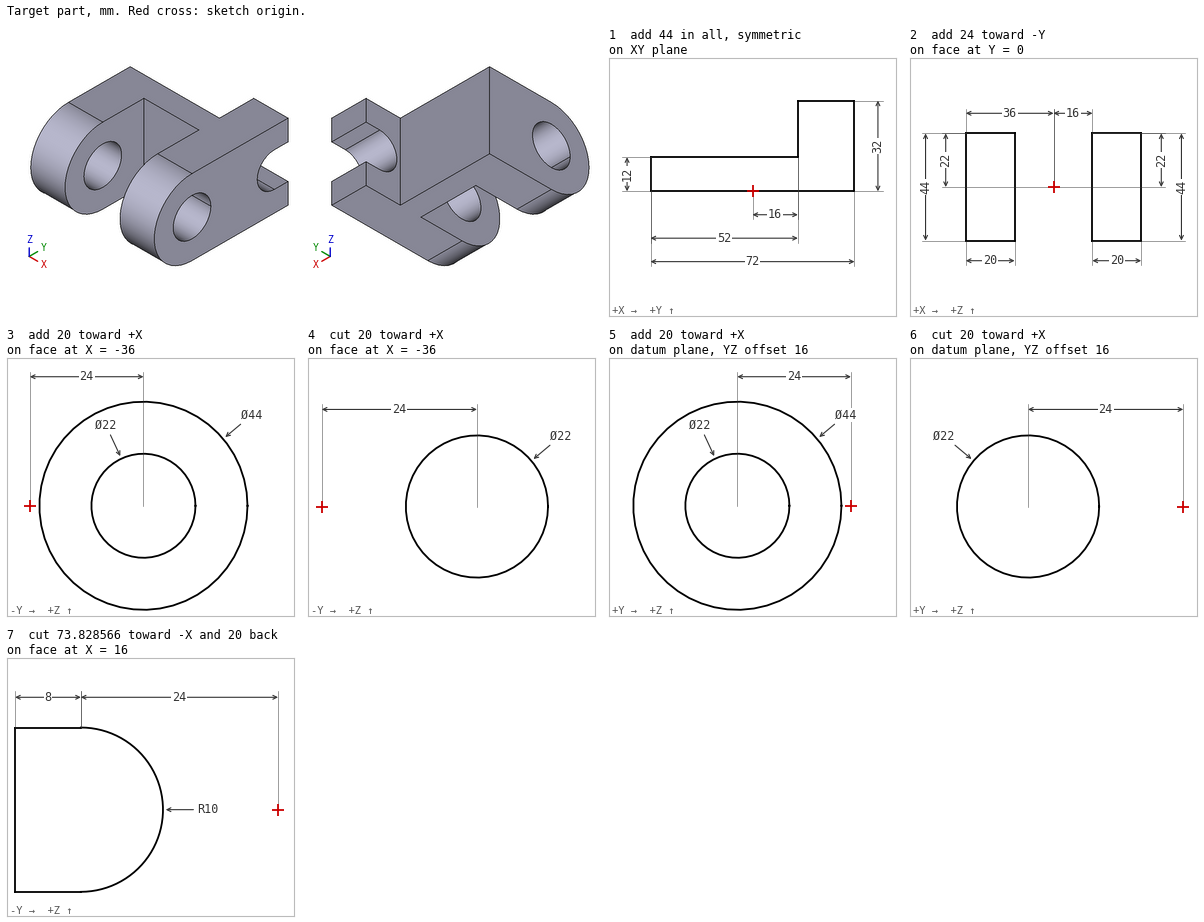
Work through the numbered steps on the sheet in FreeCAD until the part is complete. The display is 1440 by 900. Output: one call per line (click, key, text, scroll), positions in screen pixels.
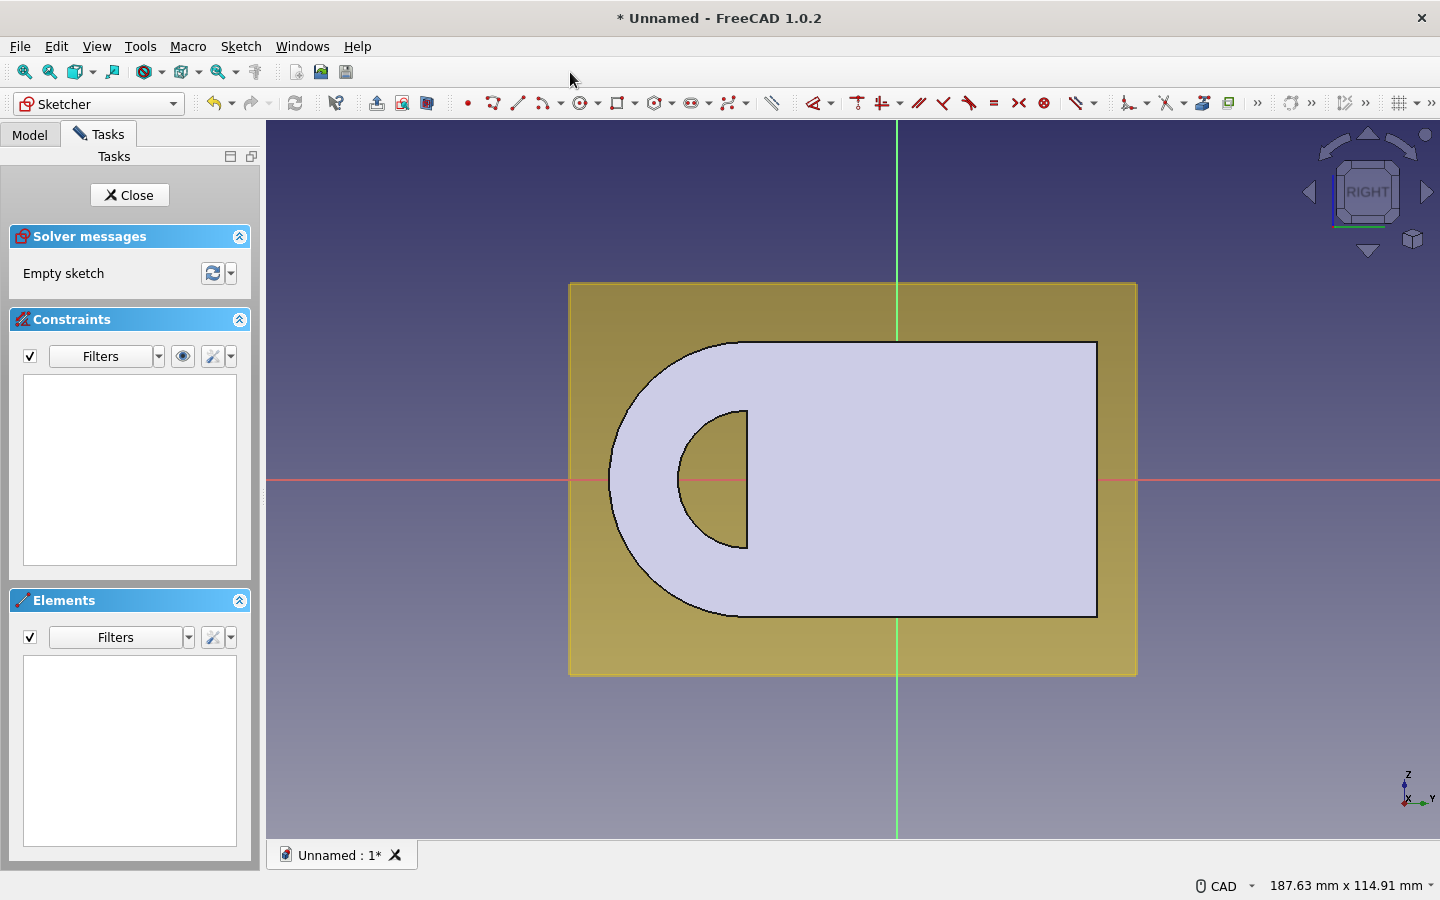
click(427, 104)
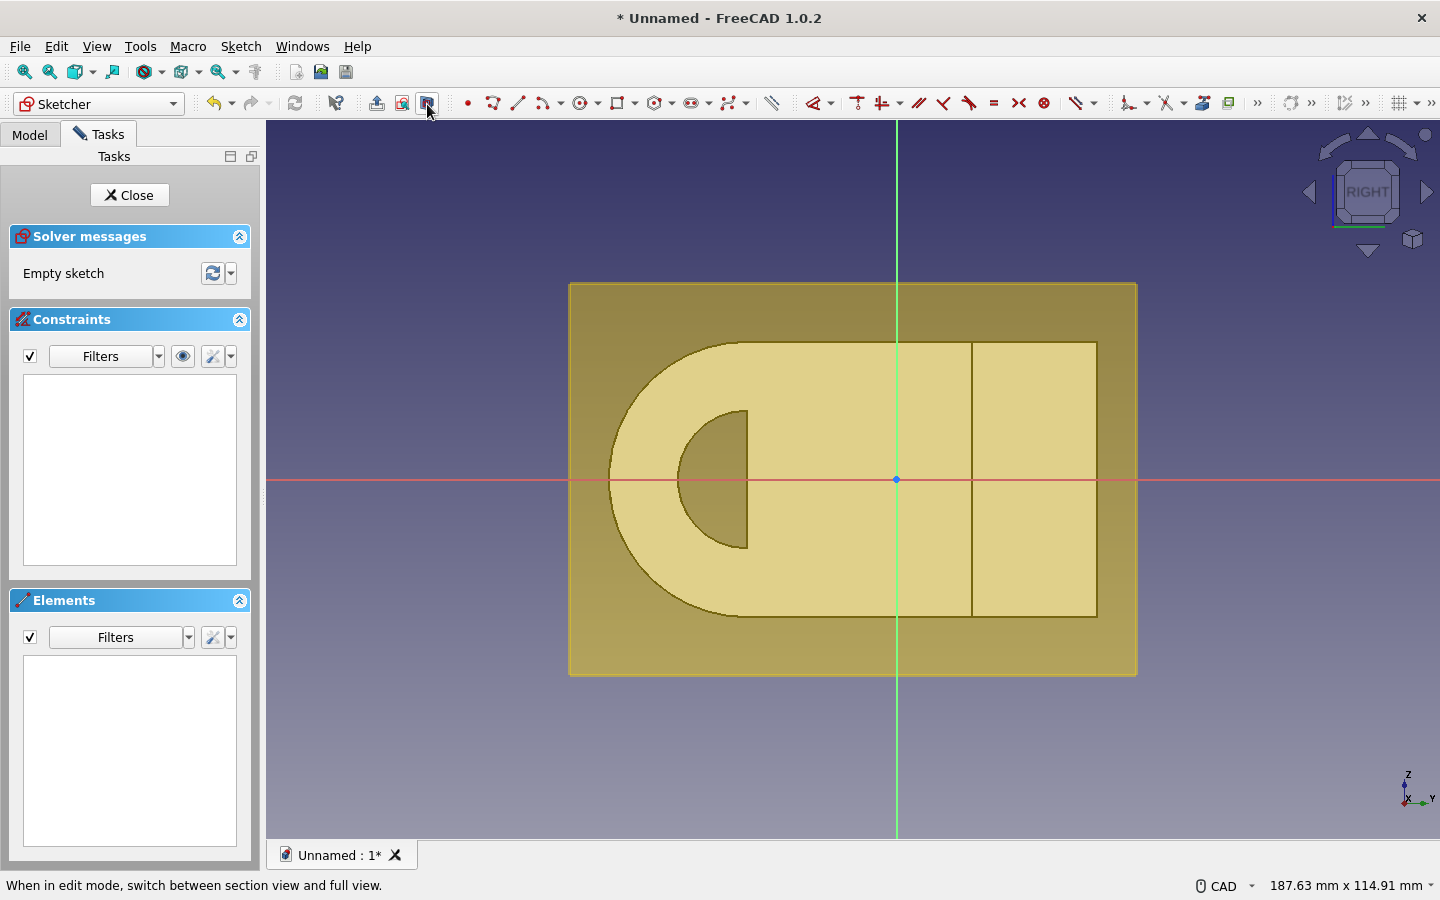
scroll(789, 480, up, 6)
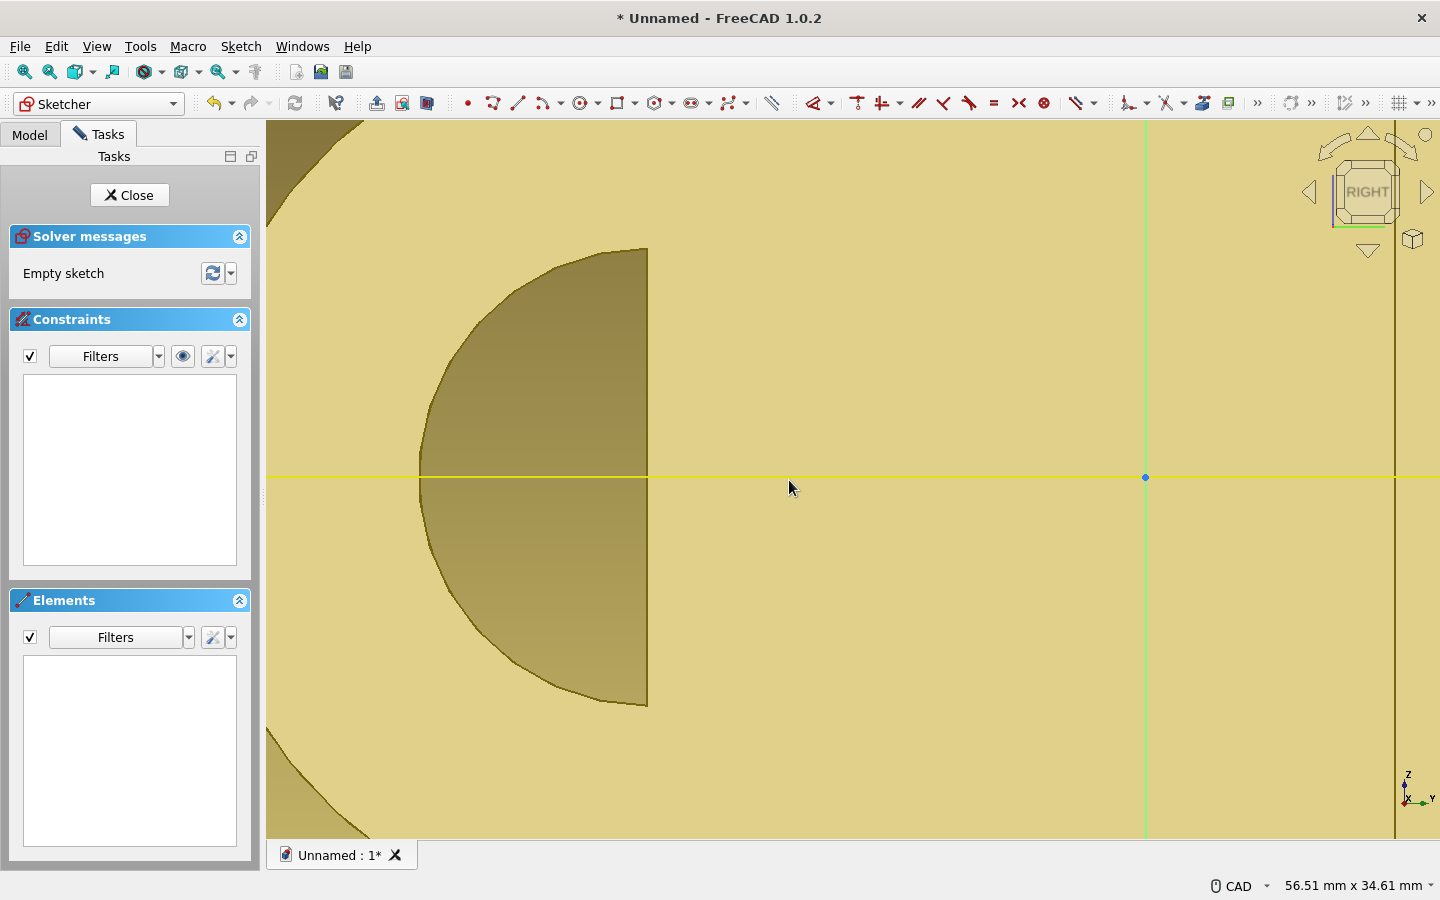
click(580, 104)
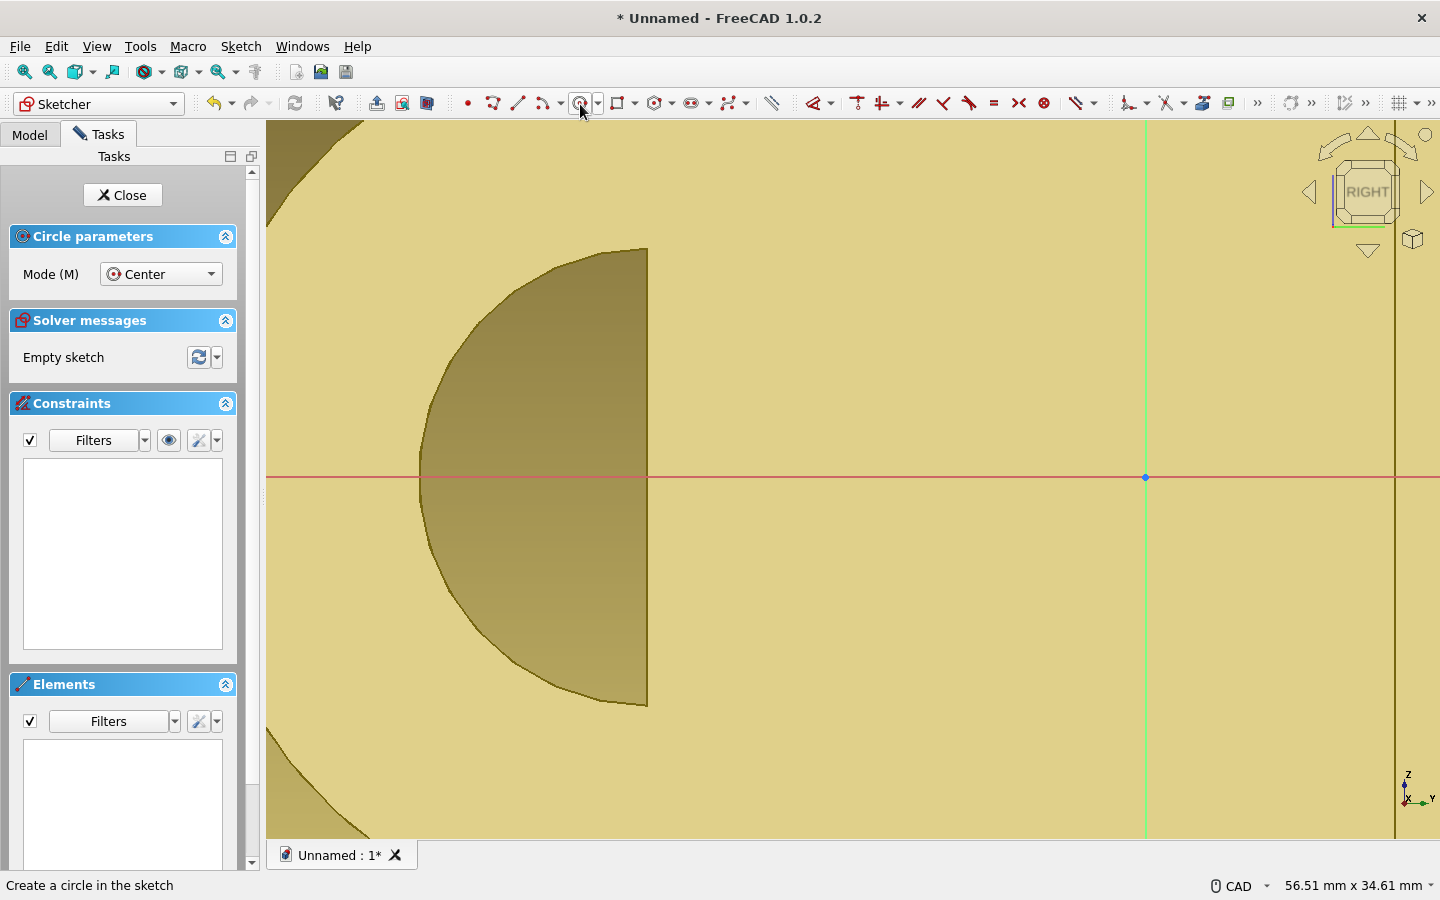
click(647, 477)
click(809, 316)
key(Escape)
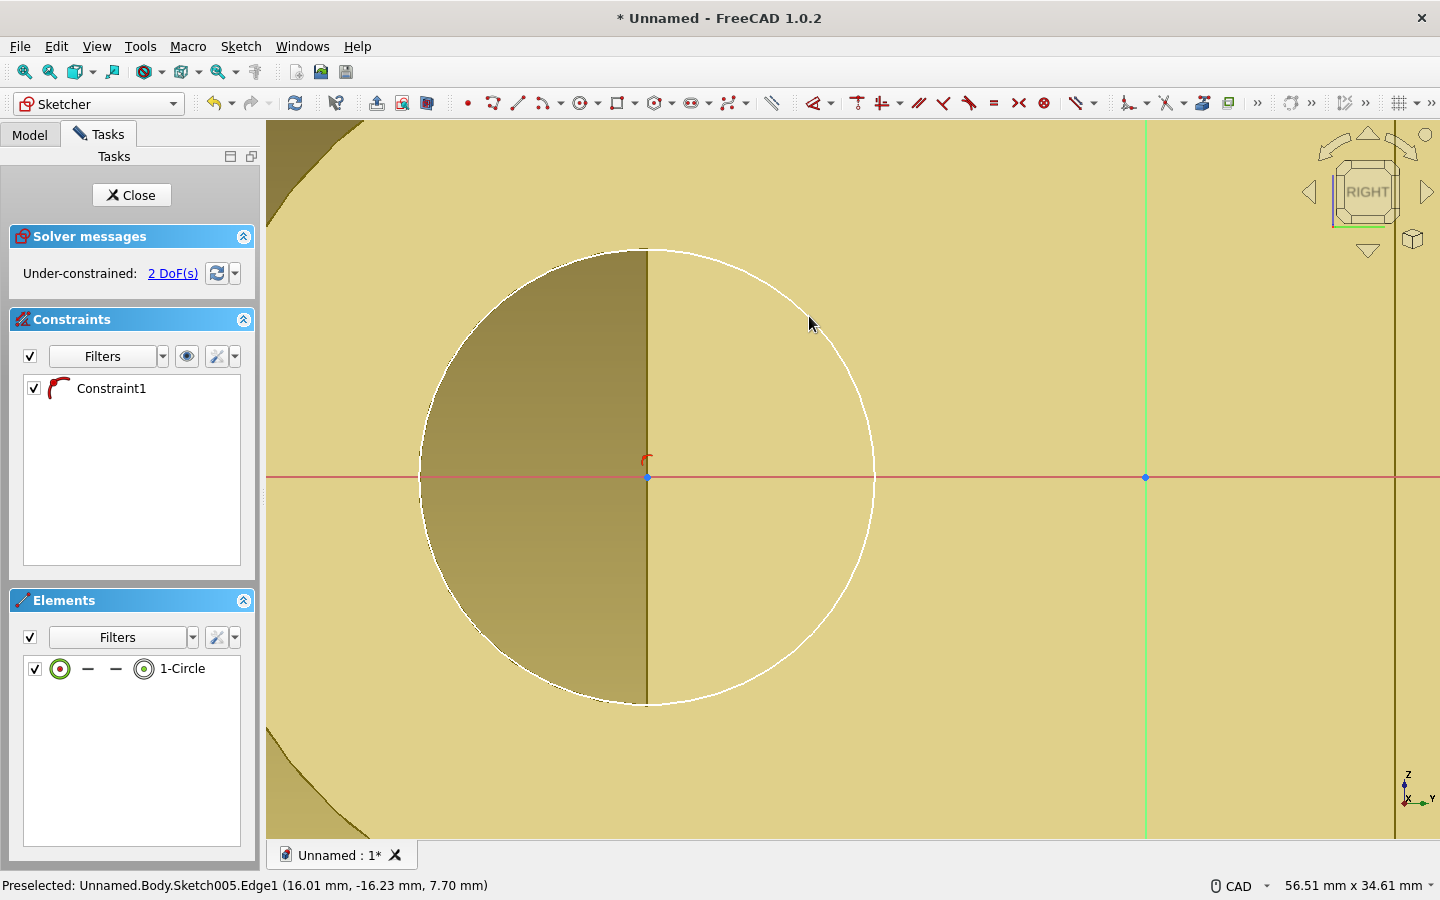
click(812, 104)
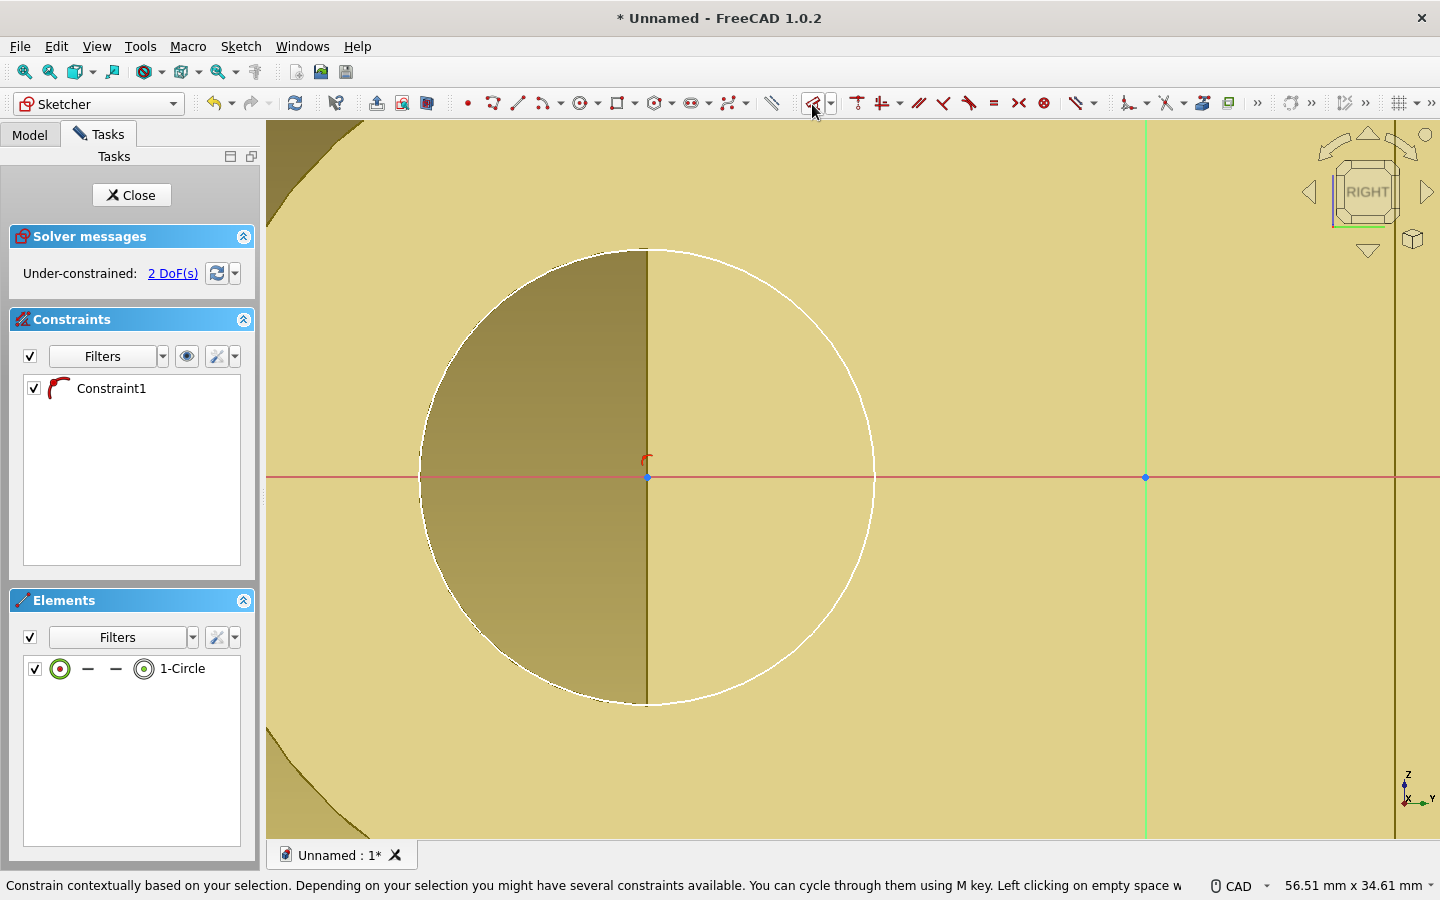
click(808, 316)
click(831, 293)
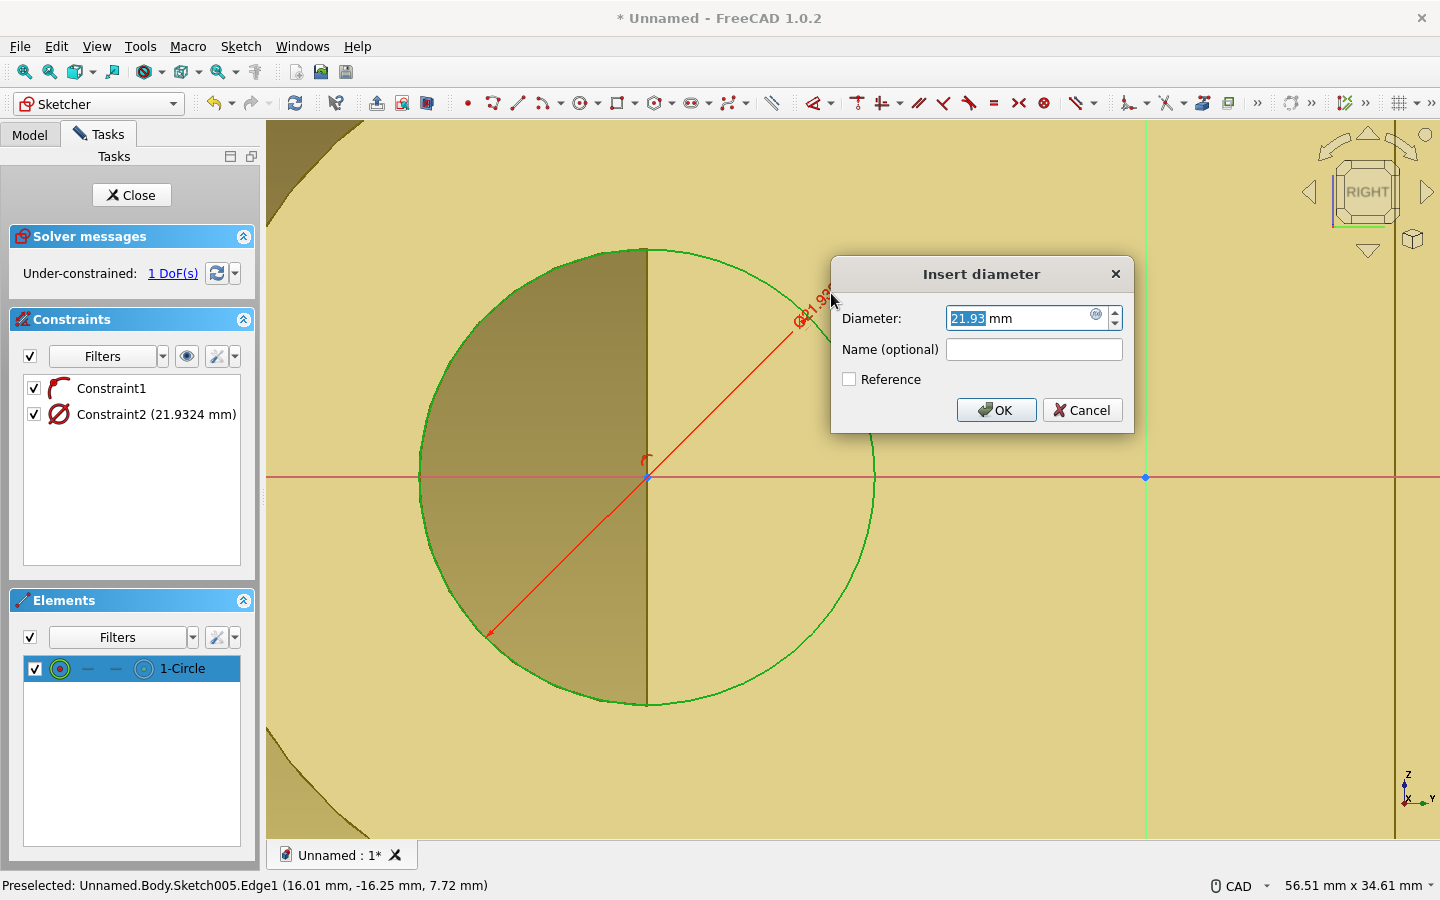
text(22)
key(Return)